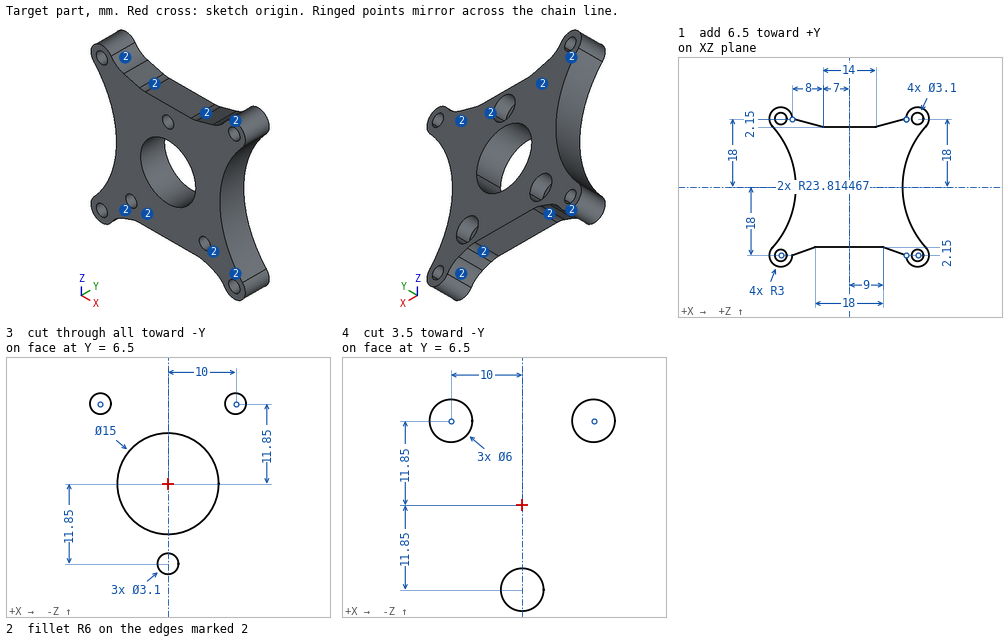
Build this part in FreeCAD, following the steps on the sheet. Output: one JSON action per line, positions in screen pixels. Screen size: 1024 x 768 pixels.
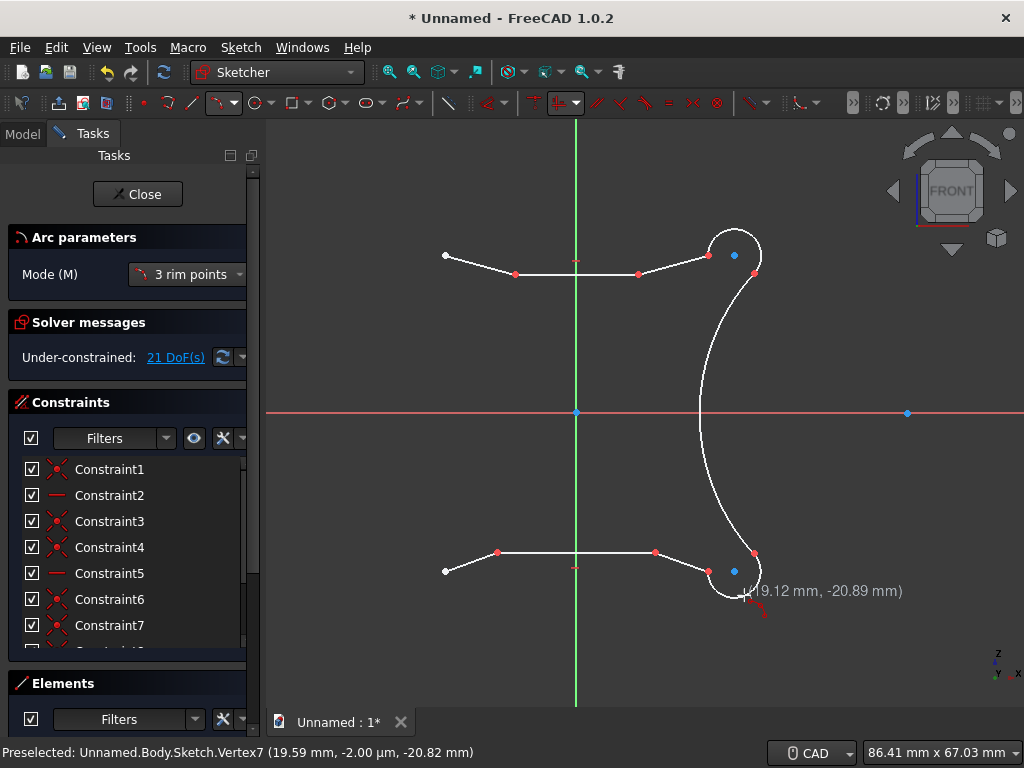
{"action": "left_click", "coordinate": [445, 572]}
{"action": "left_click", "coordinate": [399, 553]}
{"action": "left_click", "coordinate": [409, 595]}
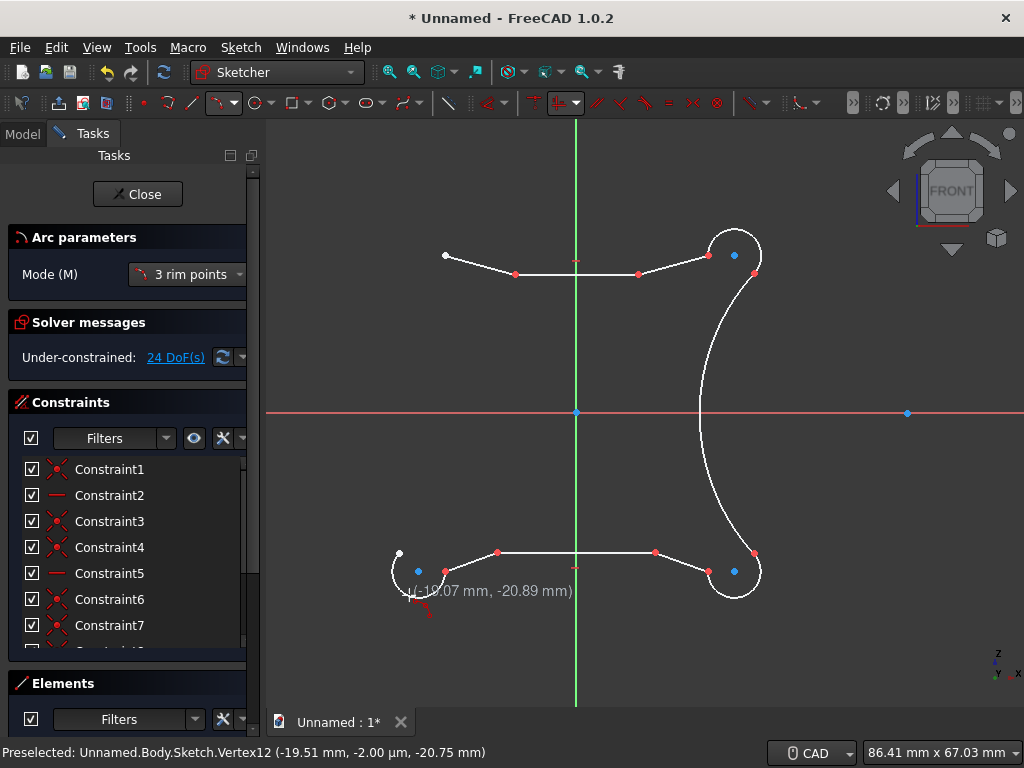
{"action": "left_click", "coordinate": [399, 554]}
{"action": "left_click", "coordinate": [399, 273]}
{"action": "left_click", "coordinate": [451, 443]}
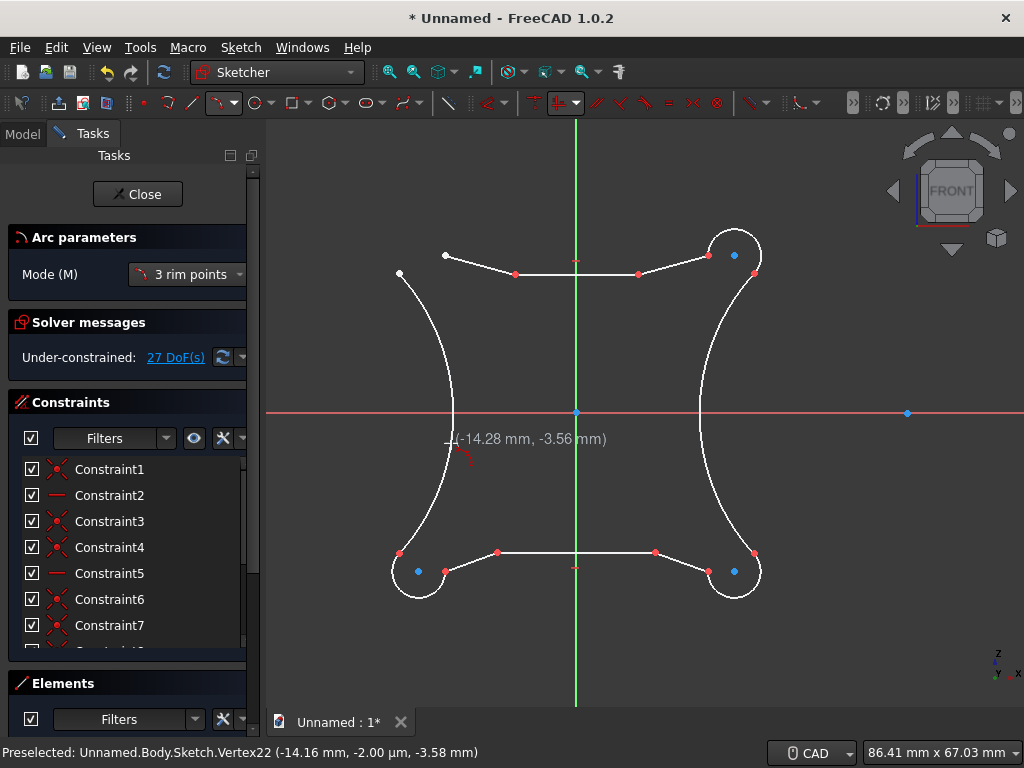
{"action": "left_click", "coordinate": [399, 274]}
{"action": "left_click", "coordinate": [445, 256]}
{"action": "left_click", "coordinate": [409, 230]}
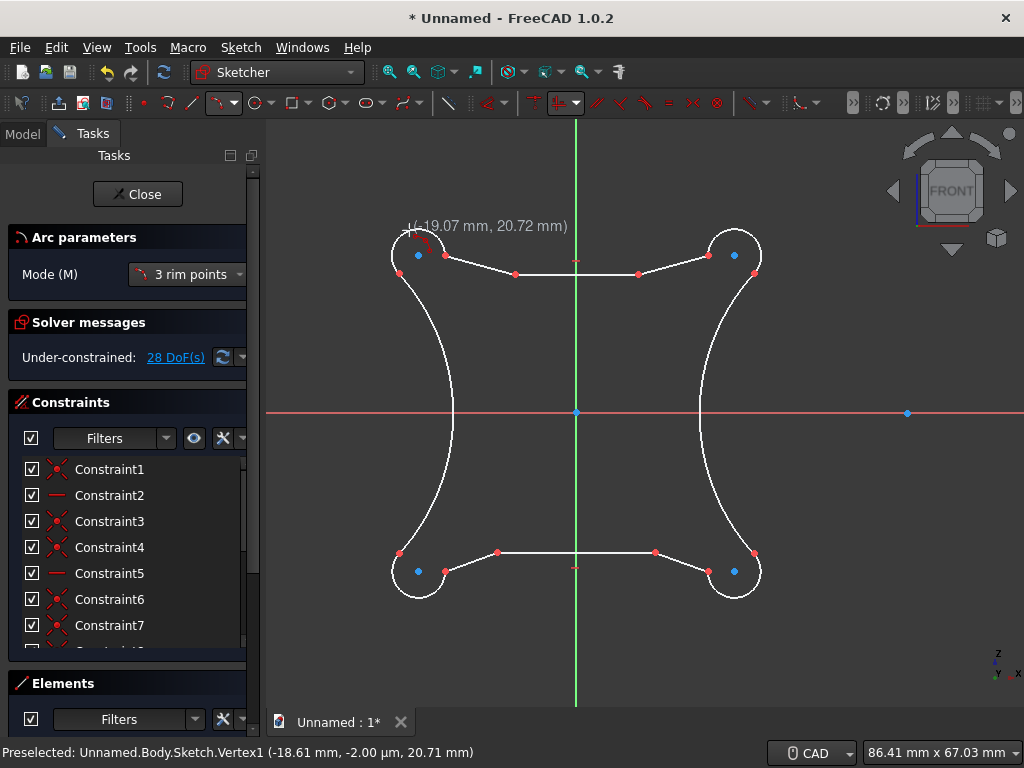
{"action": "left_click", "coordinate": [256, 104]}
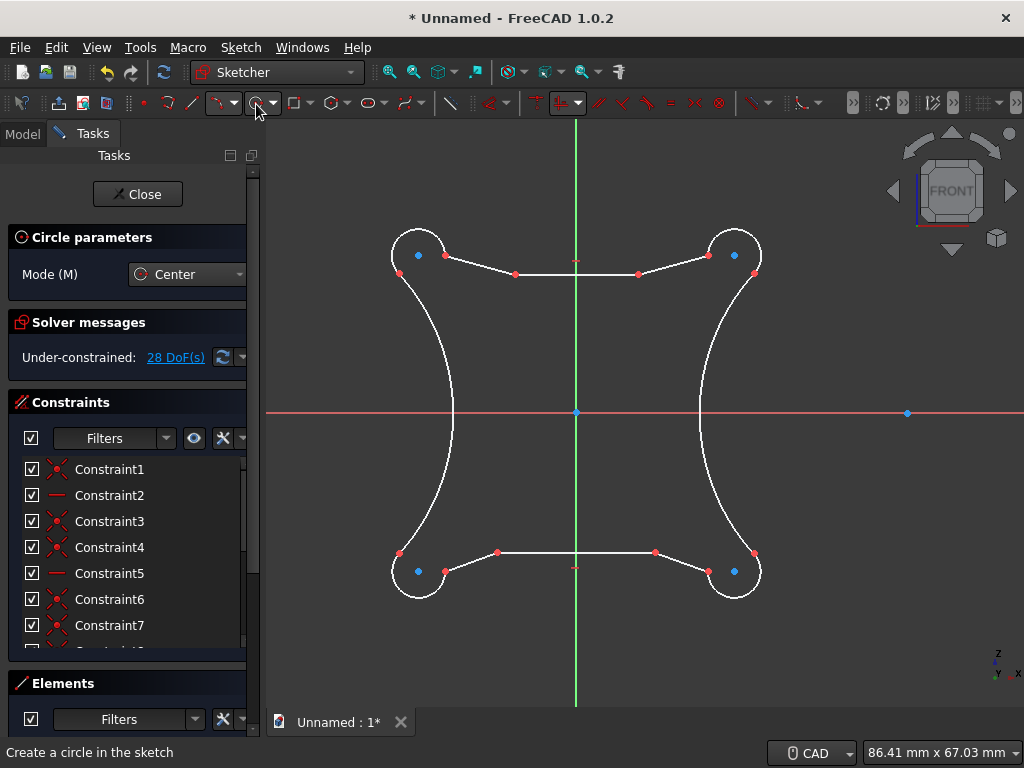
{"action": "scroll", "coordinate": [734, 255], "scroll_direction": "up", "scroll_amount": 3}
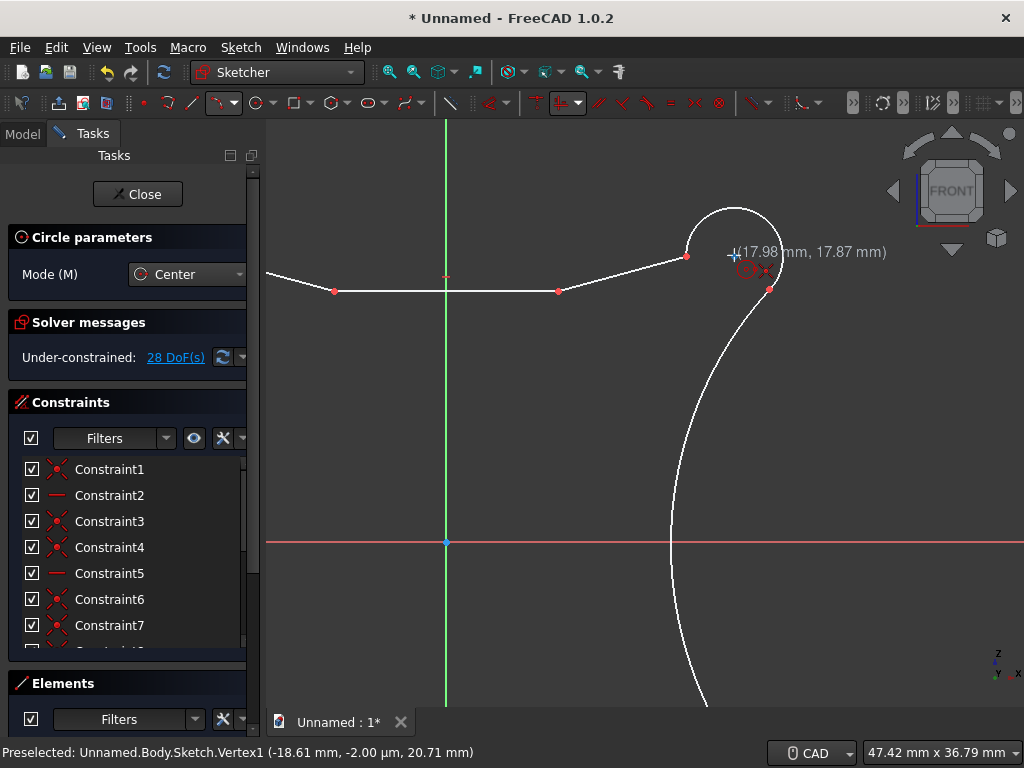
{"action": "left_click", "coordinate": [734, 255]}
{"action": "left_click", "coordinate": [751, 237]}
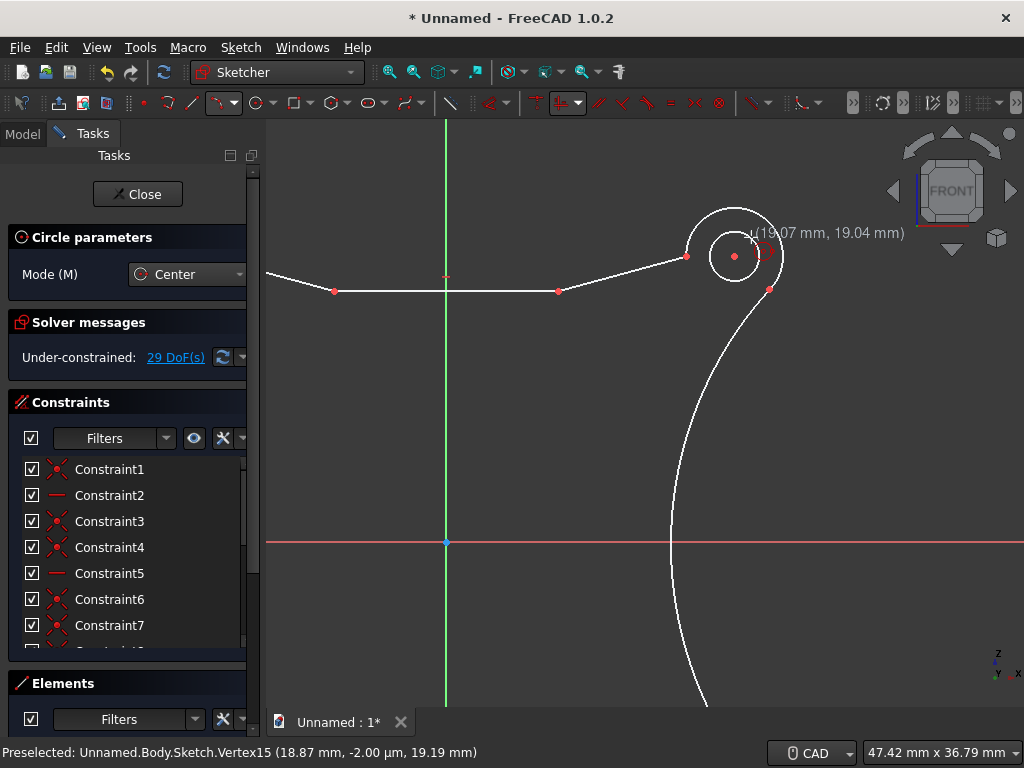
{"action": "scroll", "coordinate": [735, 256], "scroll_direction": "down", "scroll_amount": 3}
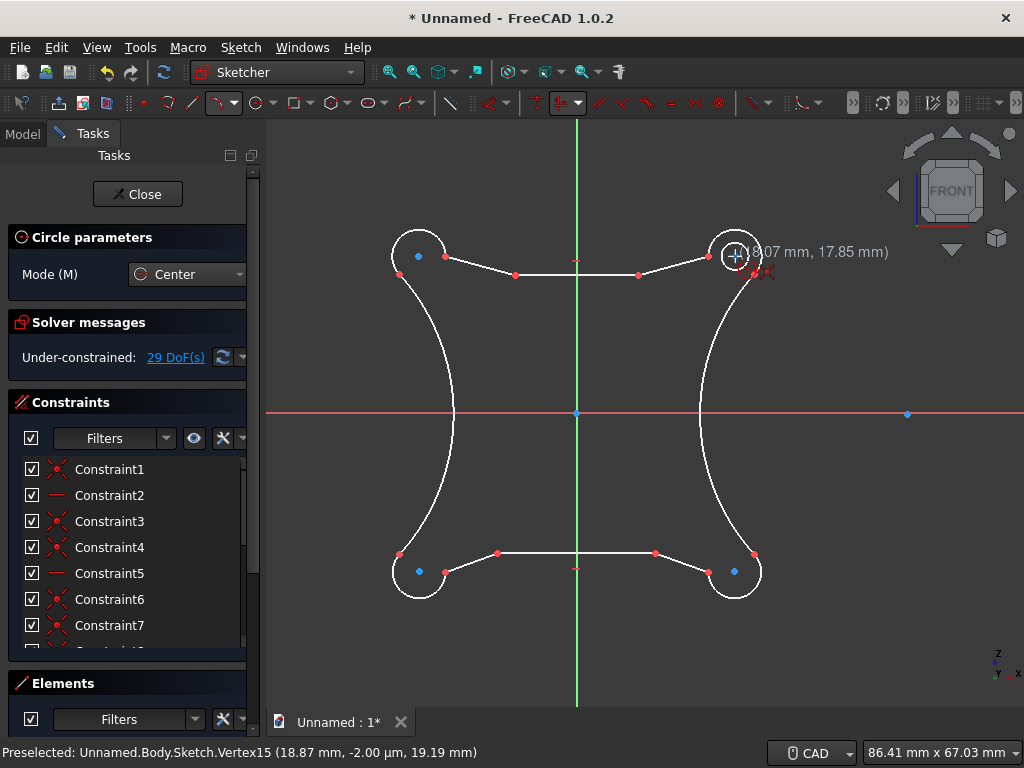
{"action": "scroll", "coordinate": [419, 255], "scroll_direction": "up", "scroll_amount": 3}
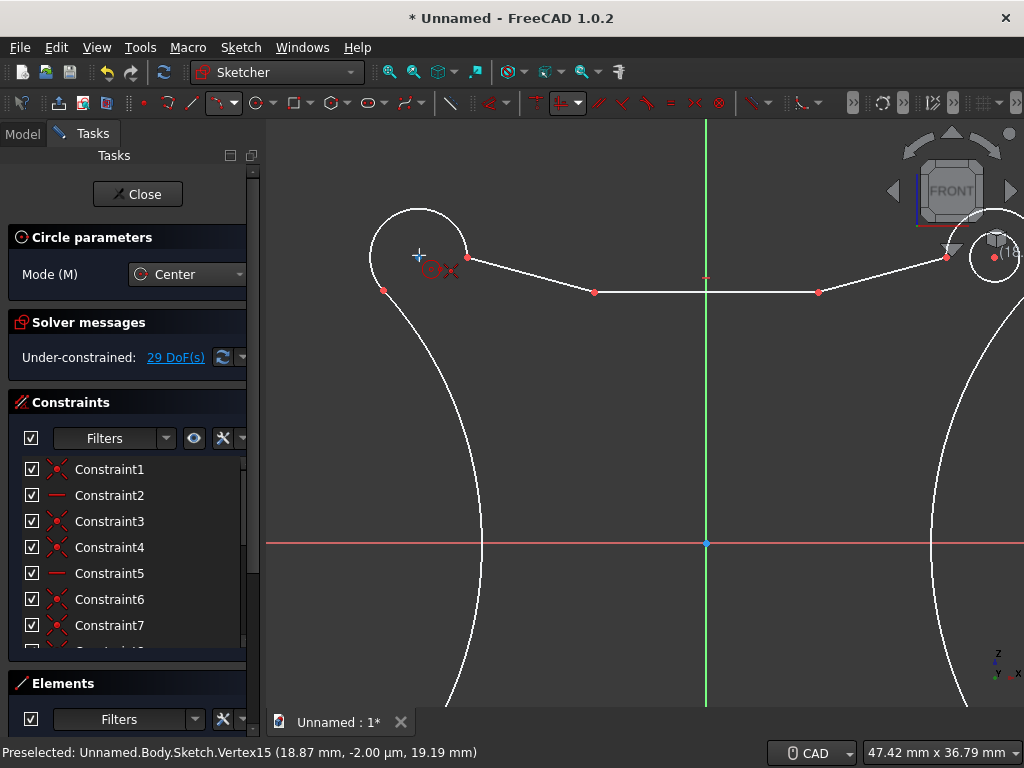
{"action": "left_click", "coordinate": [419, 255]}
{"action": "left_click", "coordinate": [436, 238]}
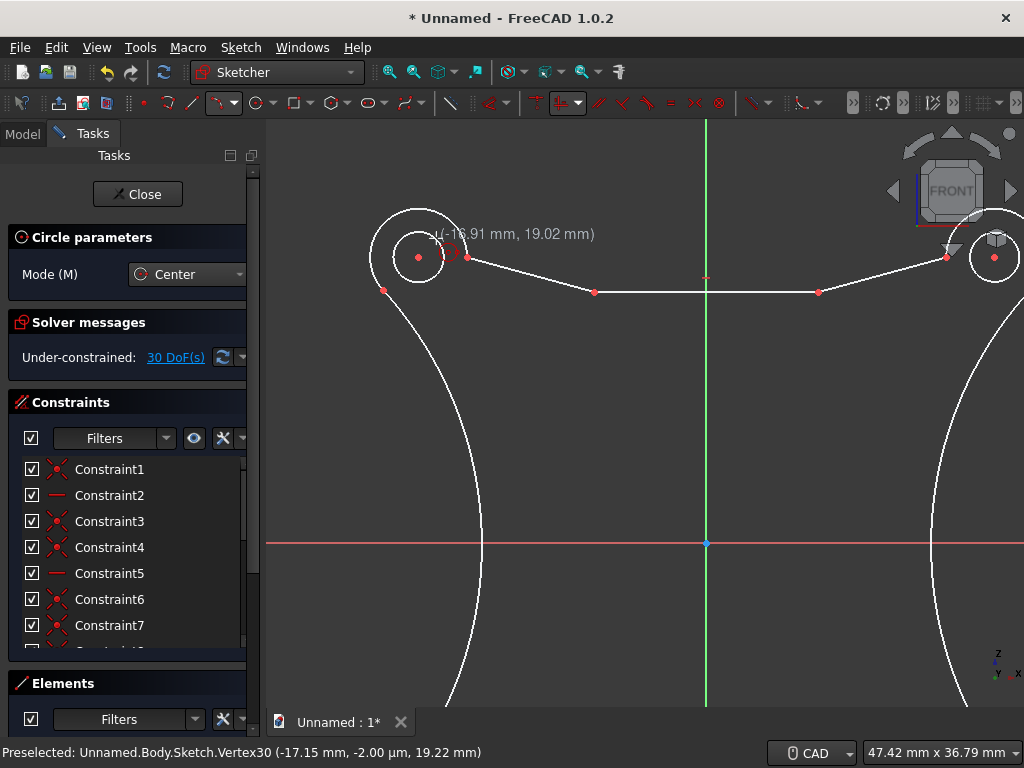
{"action": "scroll", "coordinate": [419, 255], "scroll_direction": "down", "scroll_amount": 3}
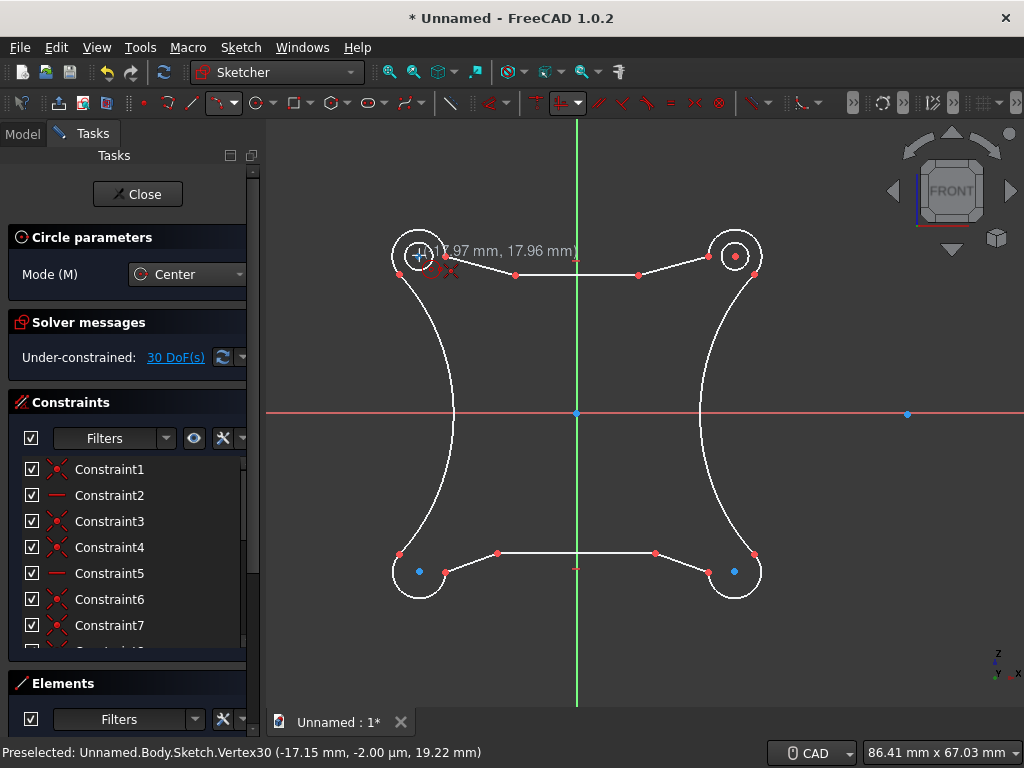
{"action": "scroll", "coordinate": [735, 571], "scroll_direction": "up", "scroll_amount": 3}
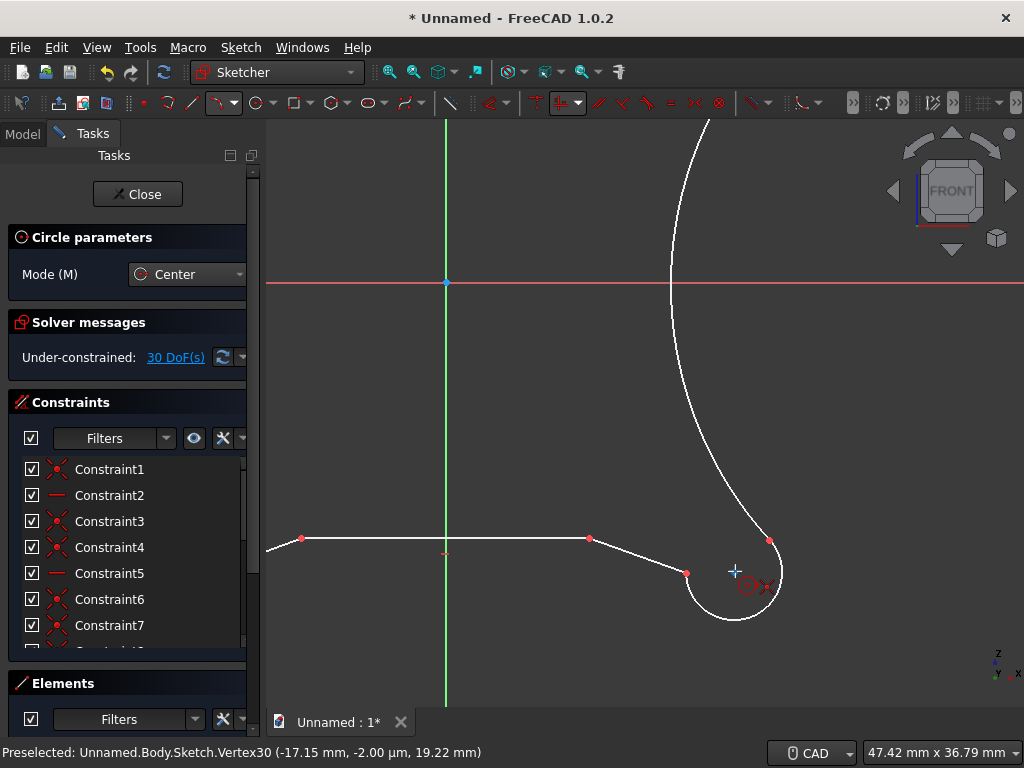
{"action": "left_click", "coordinate": [734, 571]}
{"action": "left_click", "coordinate": [751, 553]}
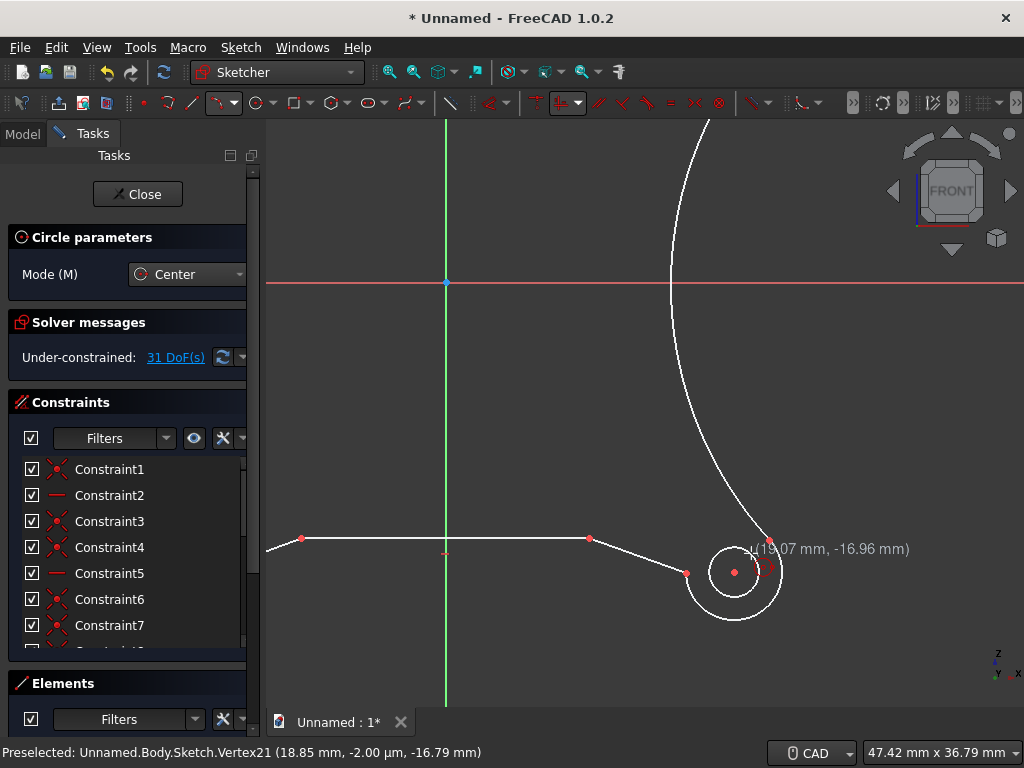
{"action": "scroll", "coordinate": [735, 571], "scroll_direction": "down", "scroll_amount": 3}